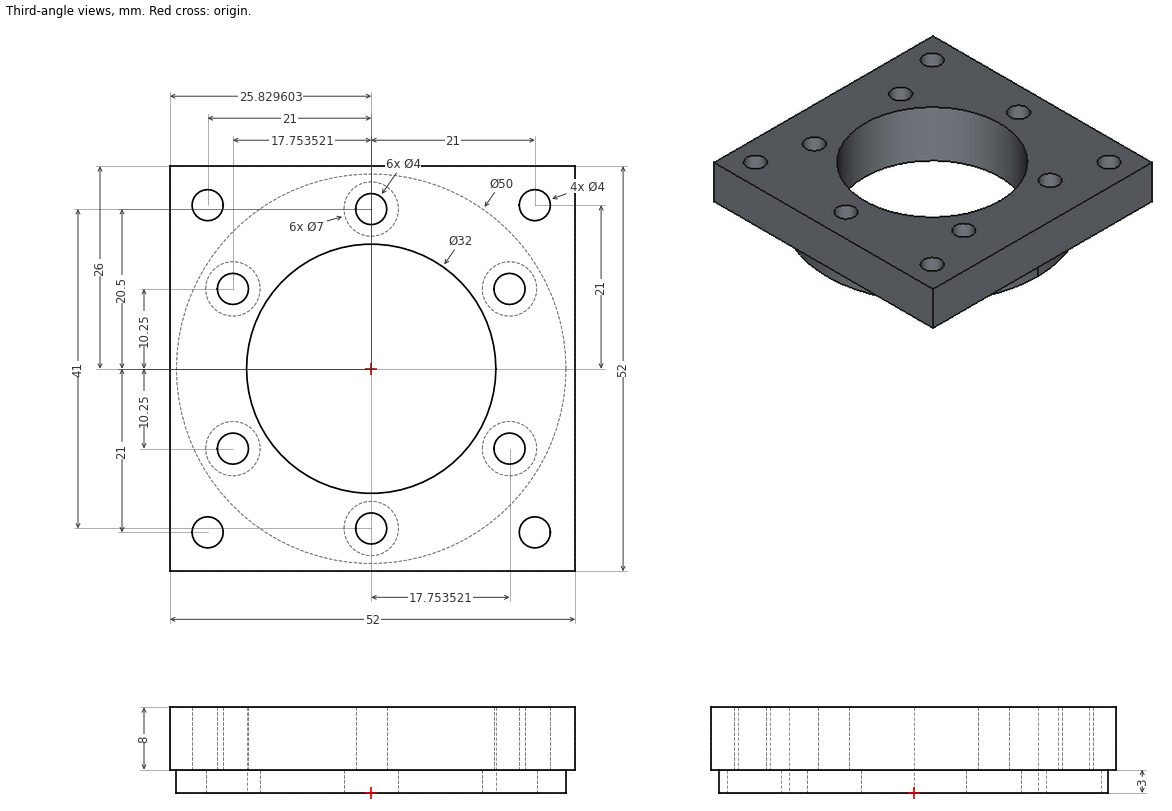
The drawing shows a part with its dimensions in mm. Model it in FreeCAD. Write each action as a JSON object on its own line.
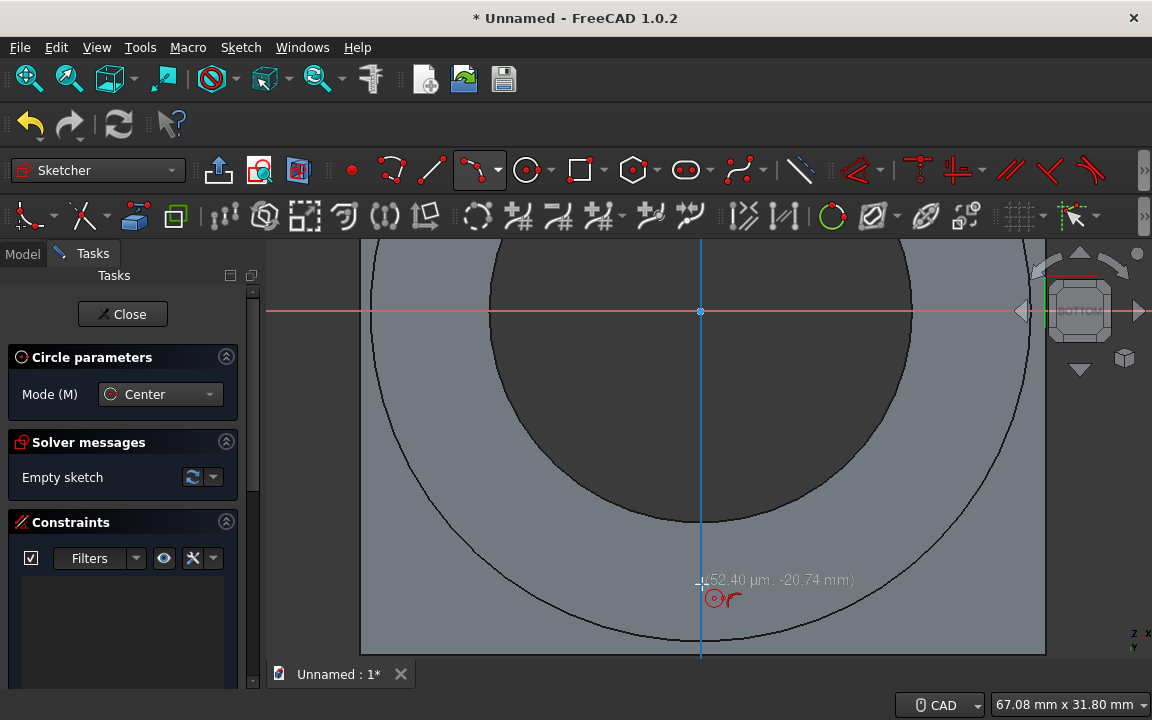
{"action": "left_click", "coordinate": [701, 582]}
{"action": "mouse_move", "coordinate": [719, 563]}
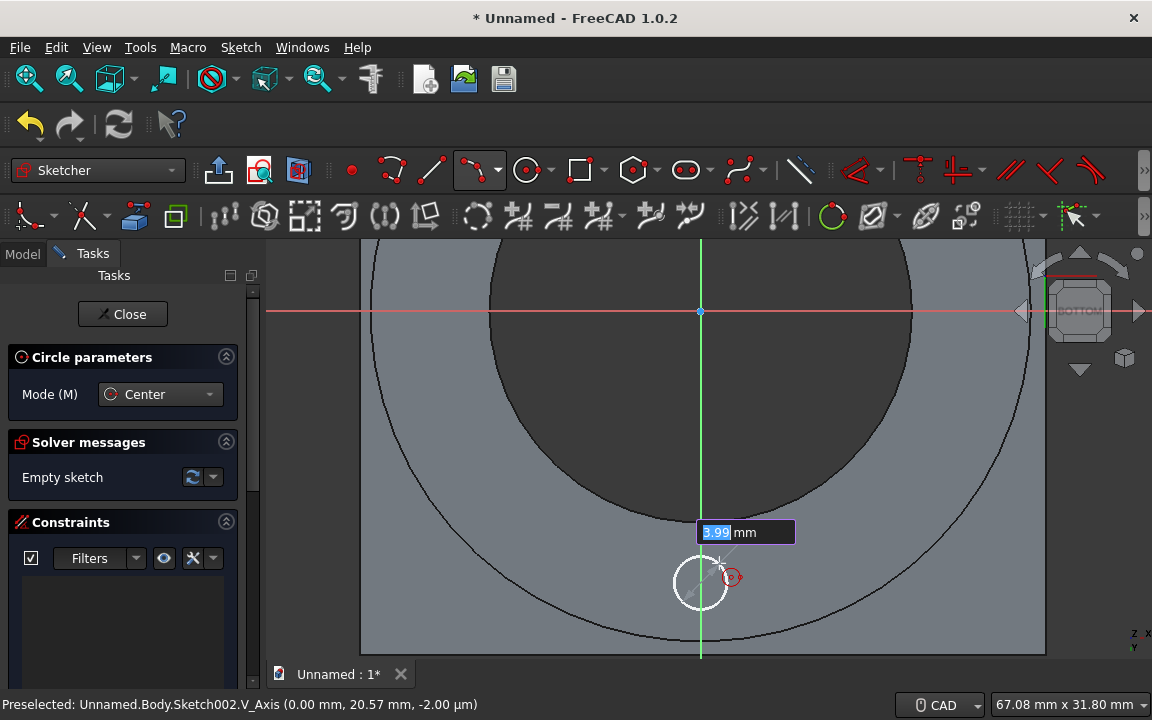
{"action": "type", "text": "4"}
{"action": "key", "text": "Return"}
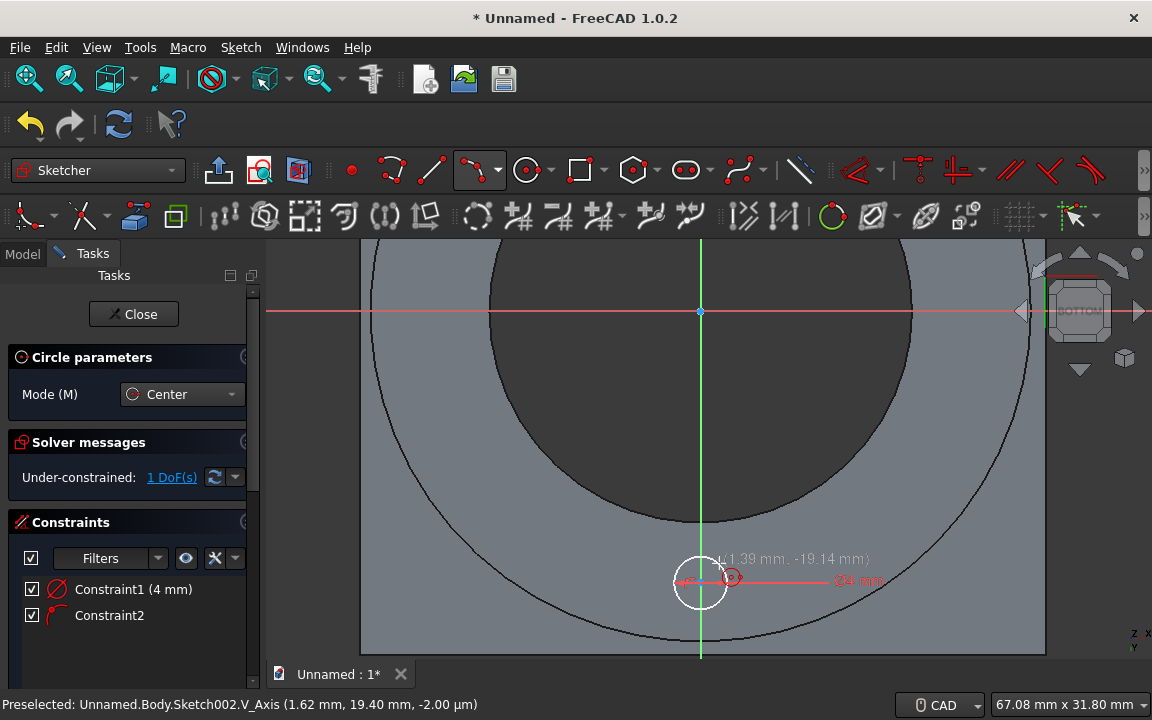
{"action": "left_click", "coordinate": [466, 447]}
{"action": "mouse_move", "coordinate": [485, 428]}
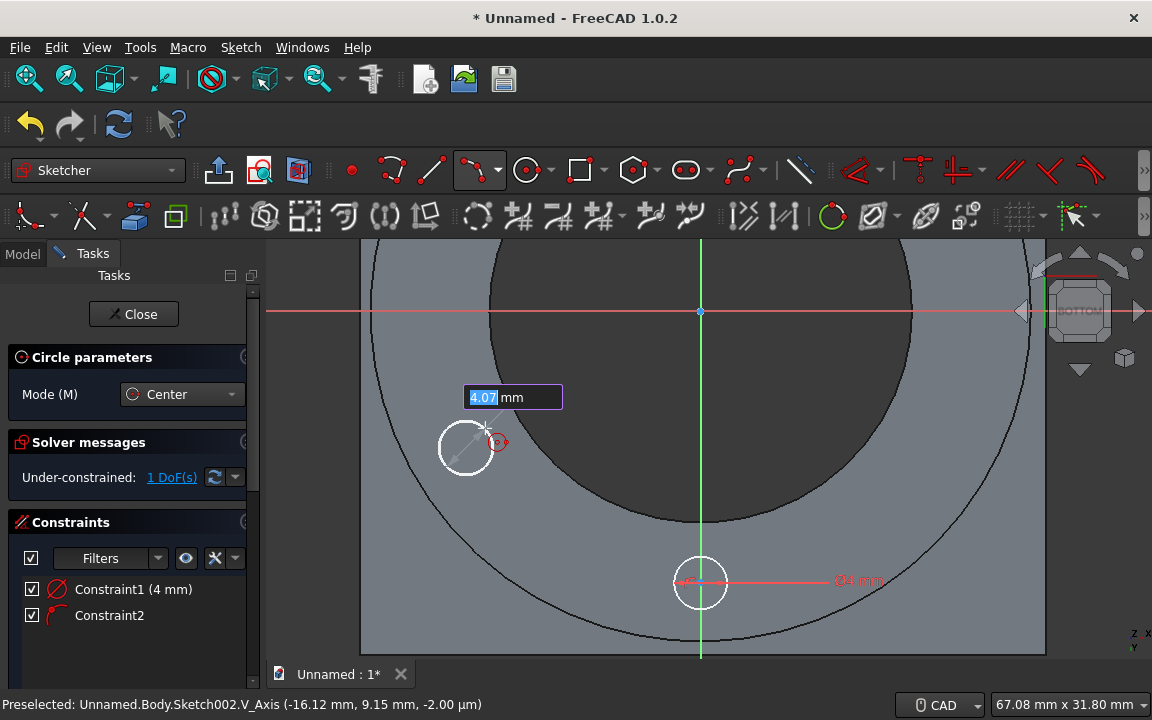
{"action": "type", "text": "4"}
{"action": "key", "text": "Return"}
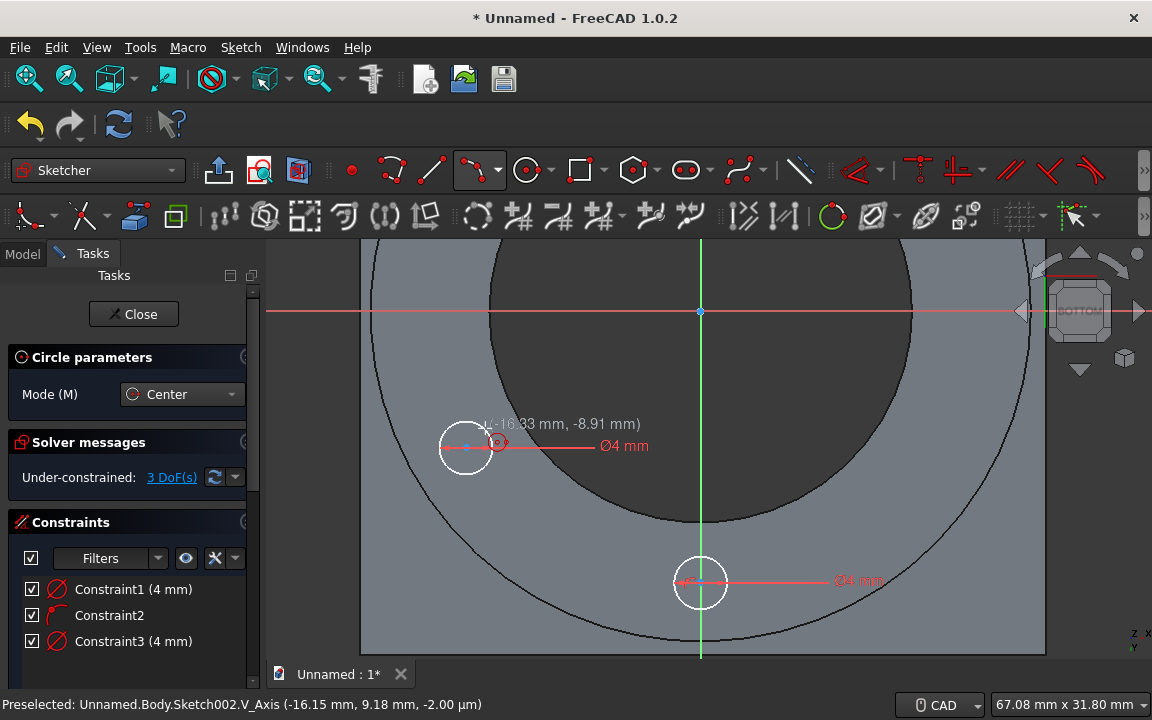
{"action": "scroll", "coordinate": [591, 561], "scroll_direction": "down", "scroll_amount": 4}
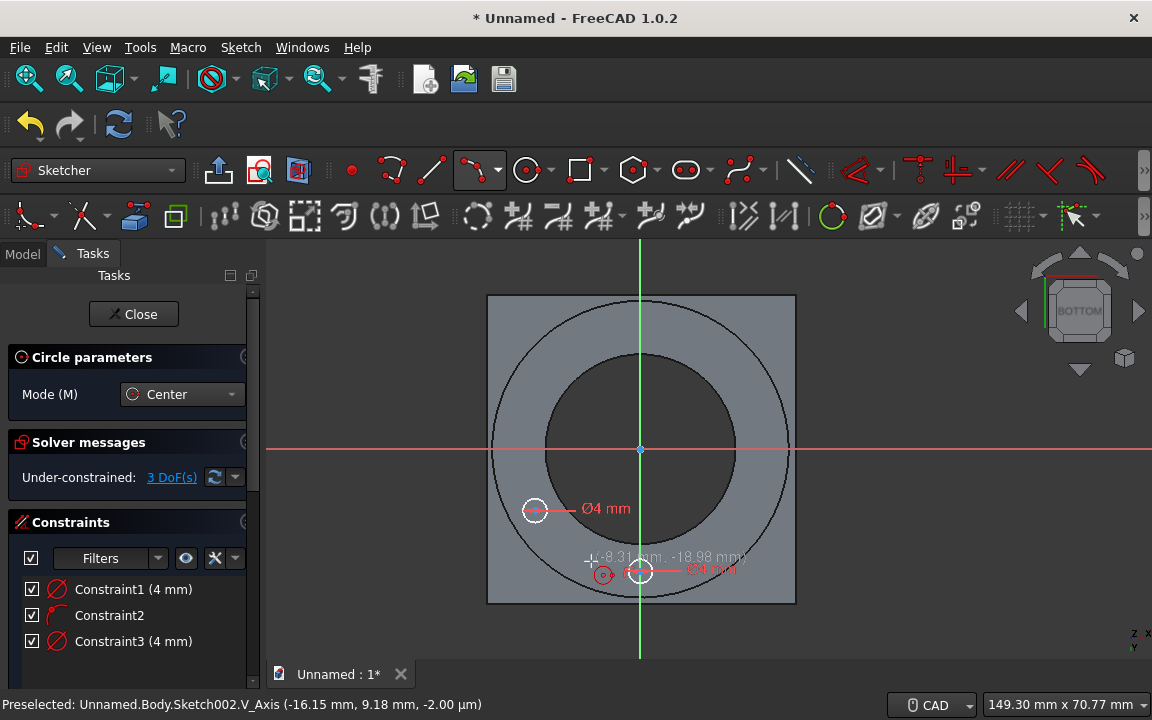
{"action": "scroll", "coordinate": [535, 388], "scroll_direction": "up", "scroll_amount": 4}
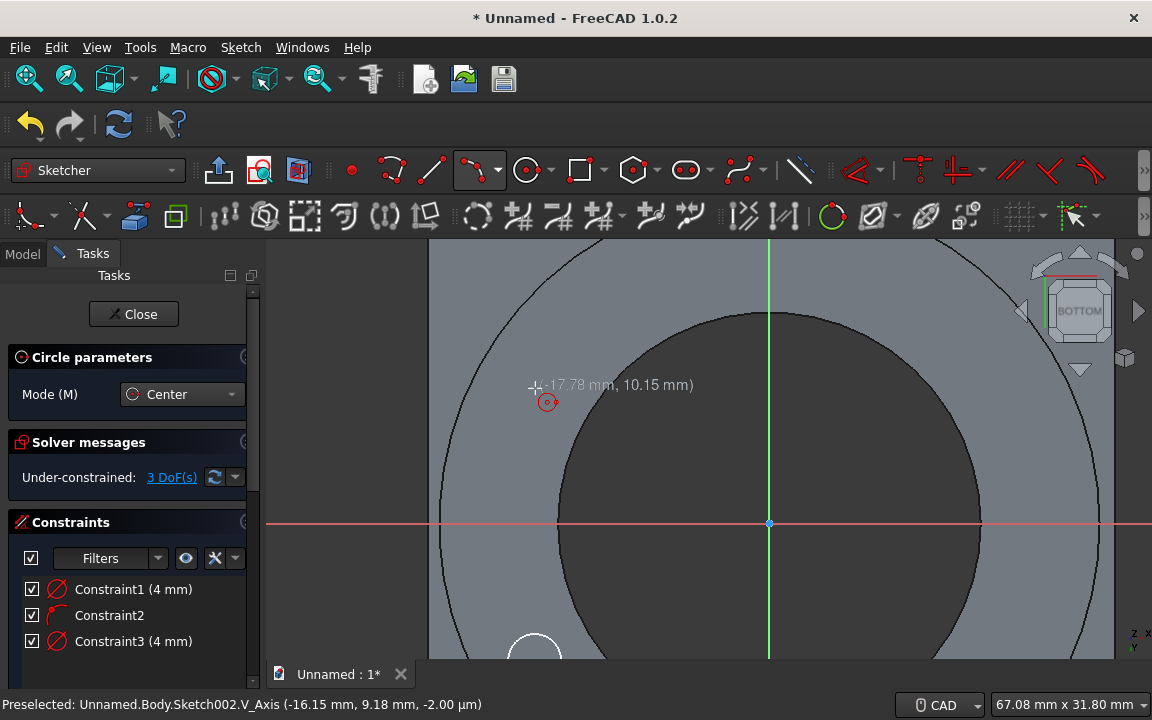
{"action": "left_click", "coordinate": [535, 388]}
{"action": "mouse_move", "coordinate": [554, 370]}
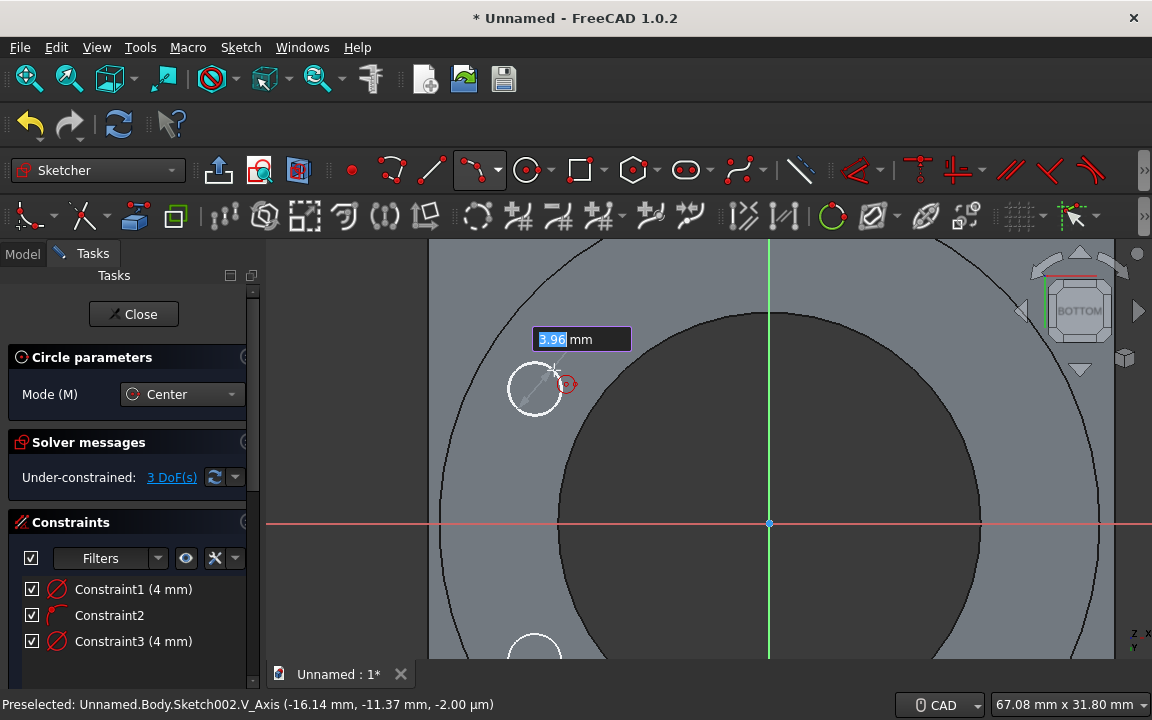
{"action": "type", "text": "4"}
{"action": "key", "text": "Return"}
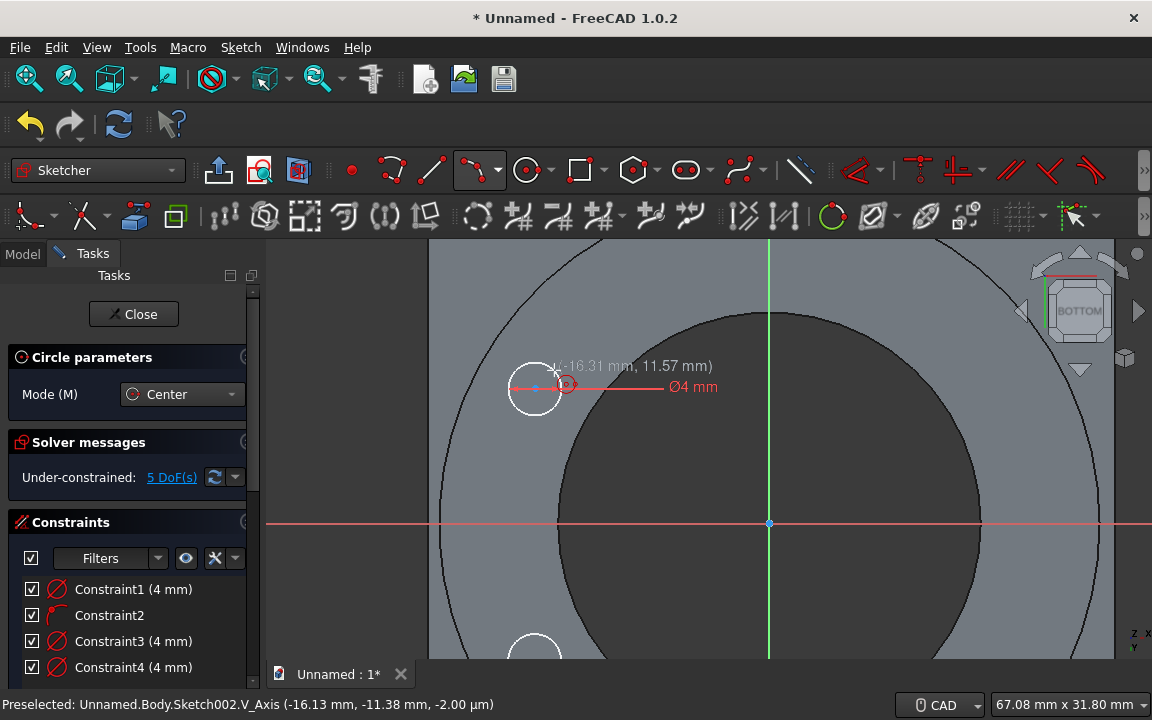
{"action": "scroll", "coordinate": [535, 388], "scroll_direction": "down", "scroll_amount": 4}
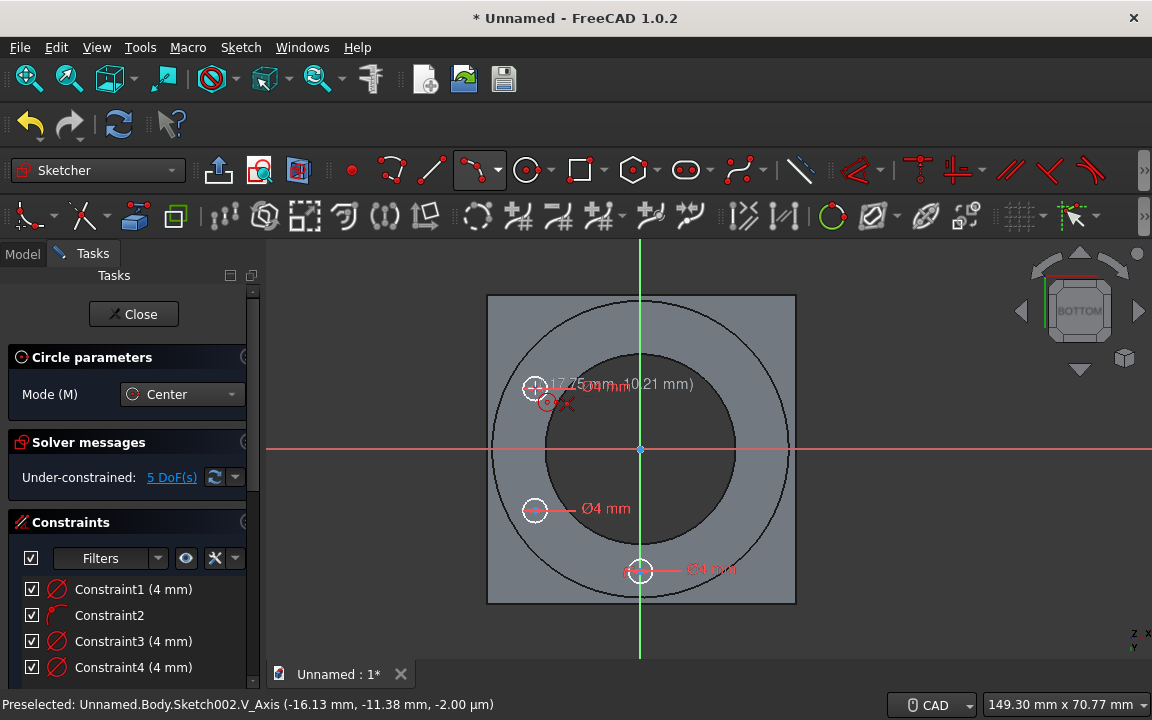
{"action": "scroll", "coordinate": [640, 328], "scroll_direction": "up", "scroll_amount": 4}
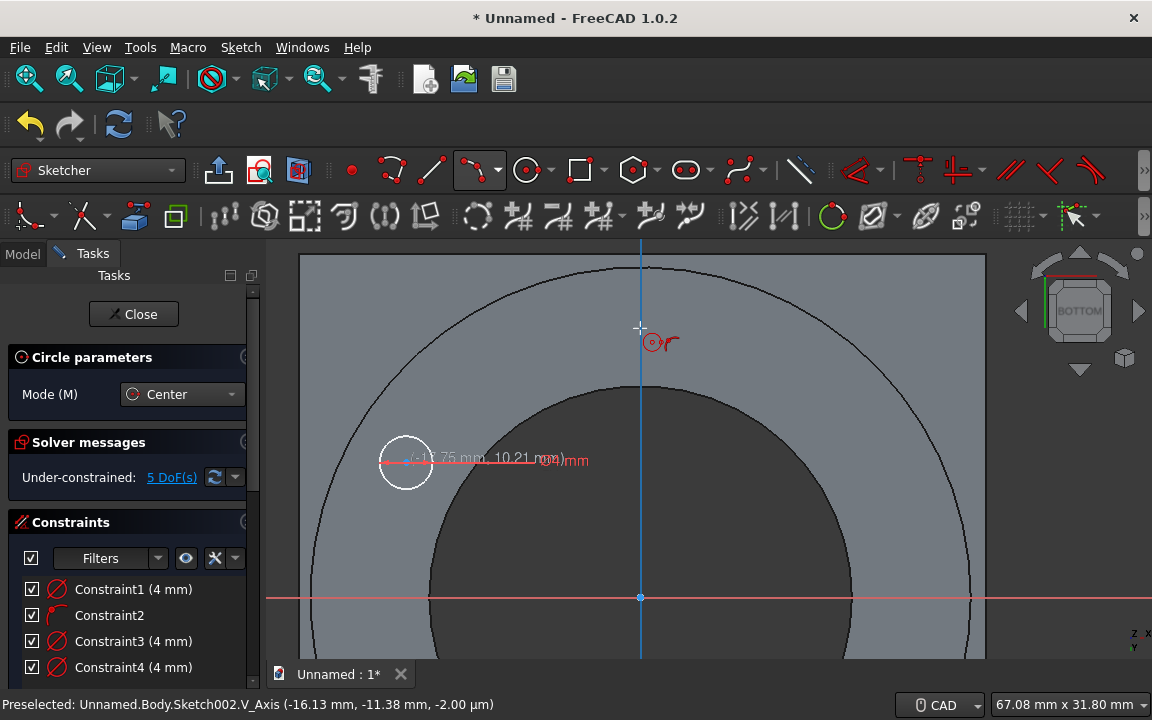
{"action": "left_click", "coordinate": [641, 327]}
{"action": "mouse_move", "coordinate": [659, 308]}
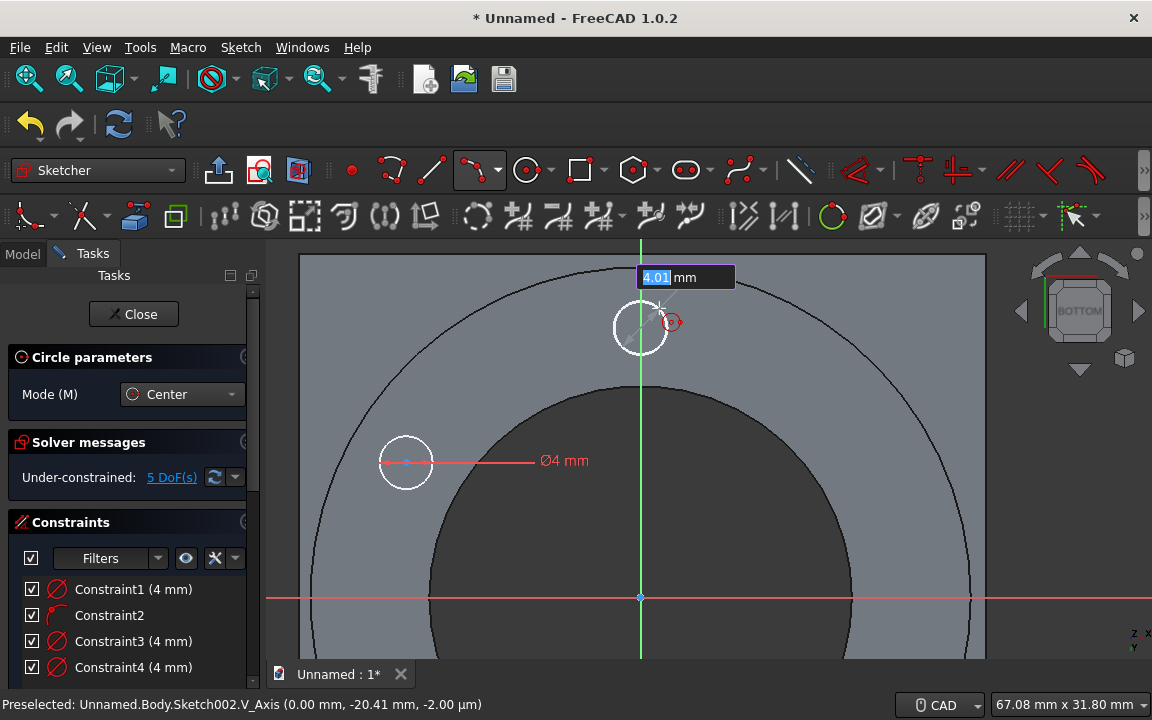
{"action": "type", "text": "4"}
{"action": "key", "text": "Return"}